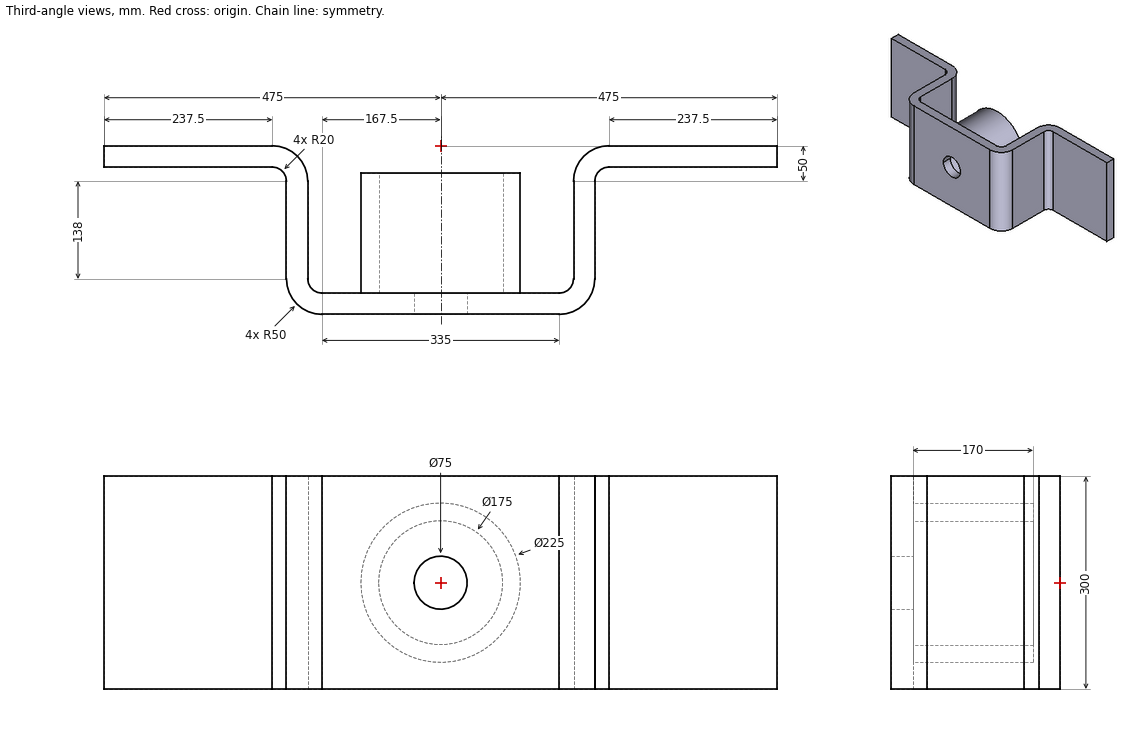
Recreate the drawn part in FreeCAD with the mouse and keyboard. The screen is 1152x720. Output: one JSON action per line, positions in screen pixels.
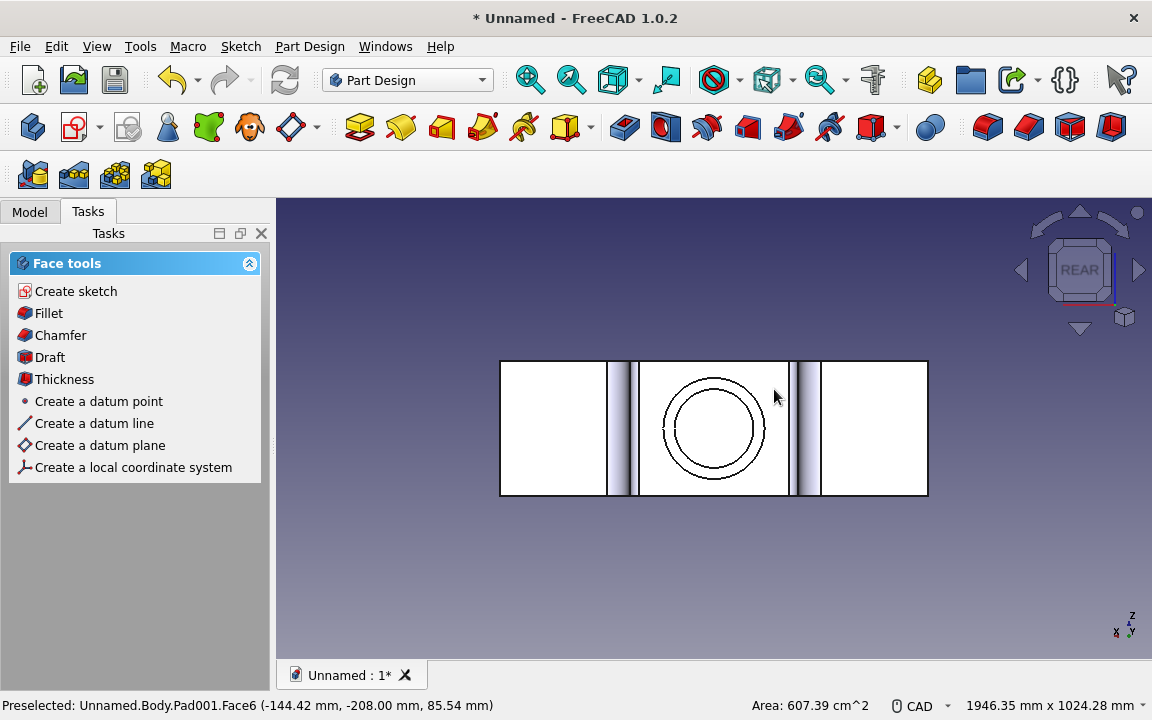
{"action": "left_click", "coordinate": [74, 128]}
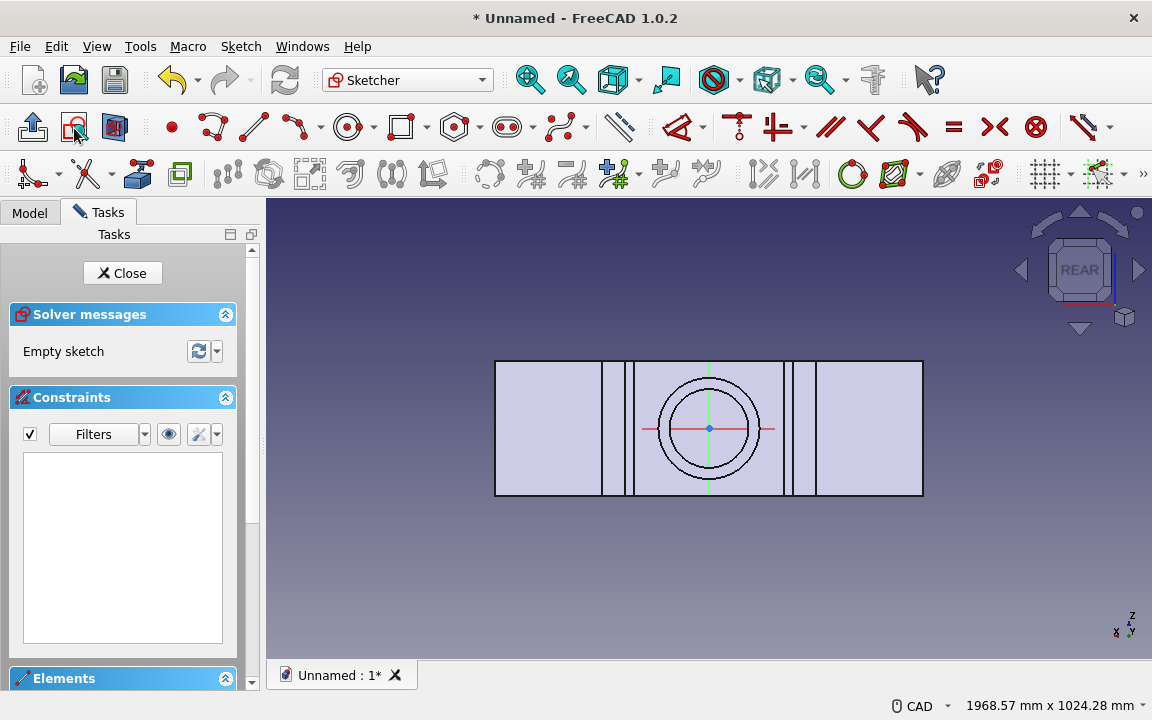
{"action": "scroll", "coordinate": [718, 429], "scroll_direction": "up", "scroll_amount": 11}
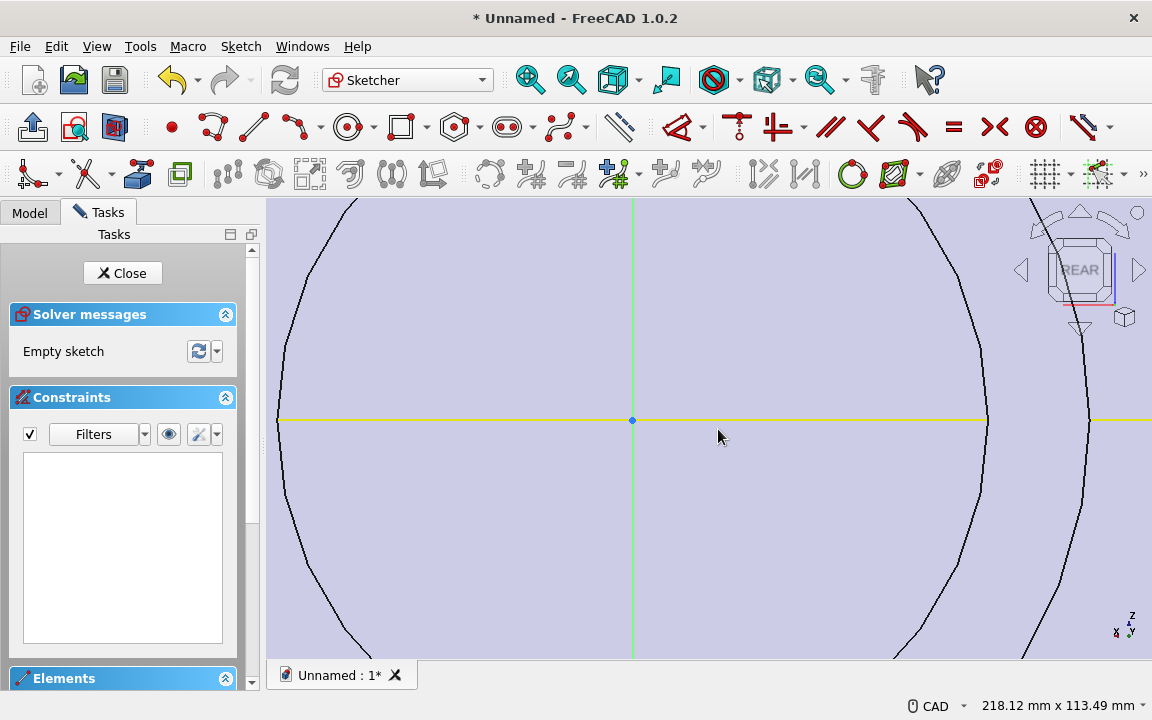
{"action": "key", "text": "g c"}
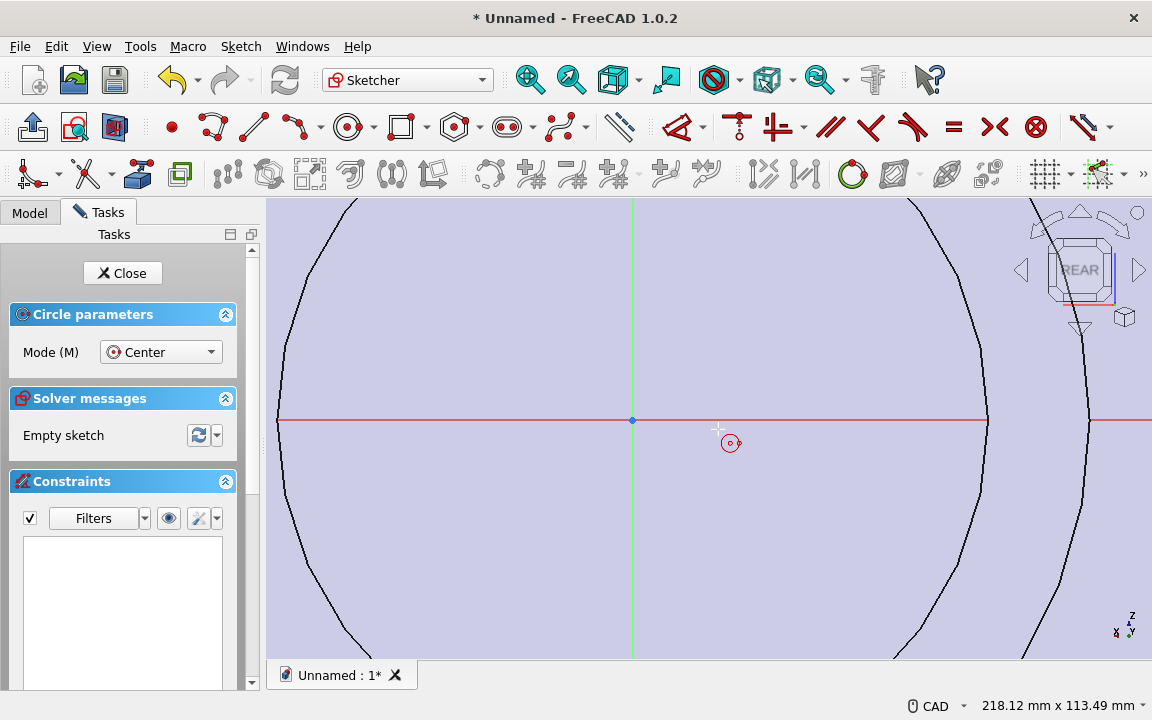
{"action": "left_click", "coordinate": [633, 420]}
{"action": "left_click", "coordinate": [740, 313]}
{"action": "key", "text": "Escape"}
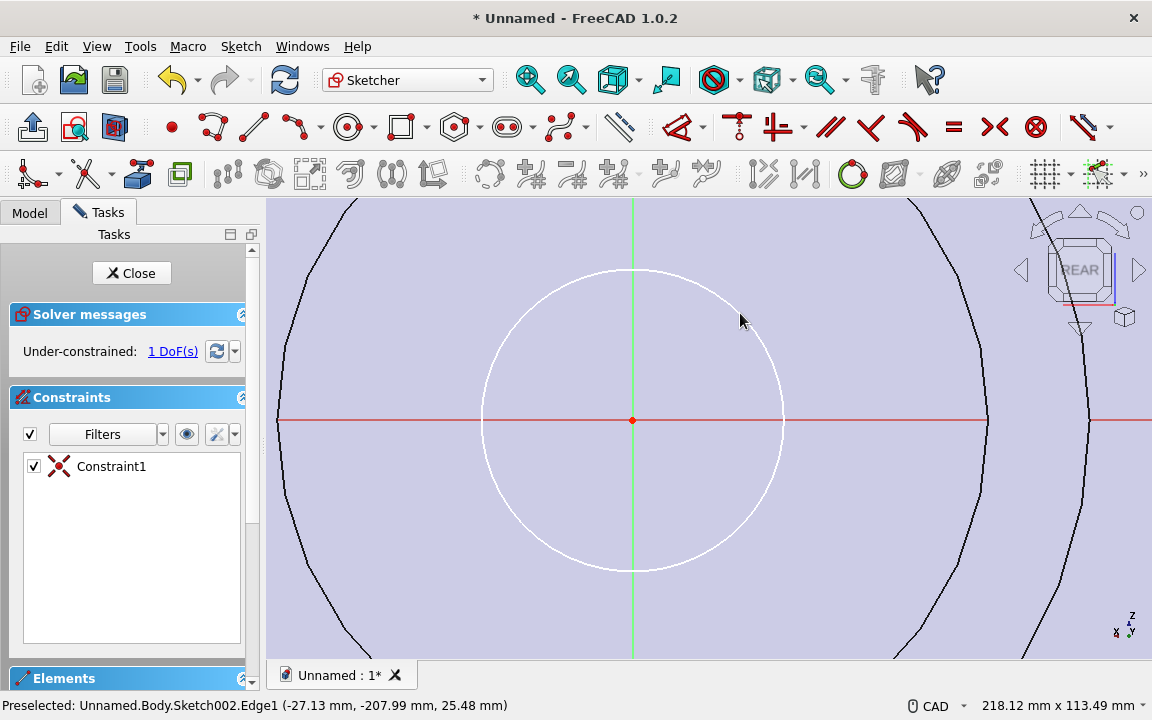
{"action": "key", "text": "d"}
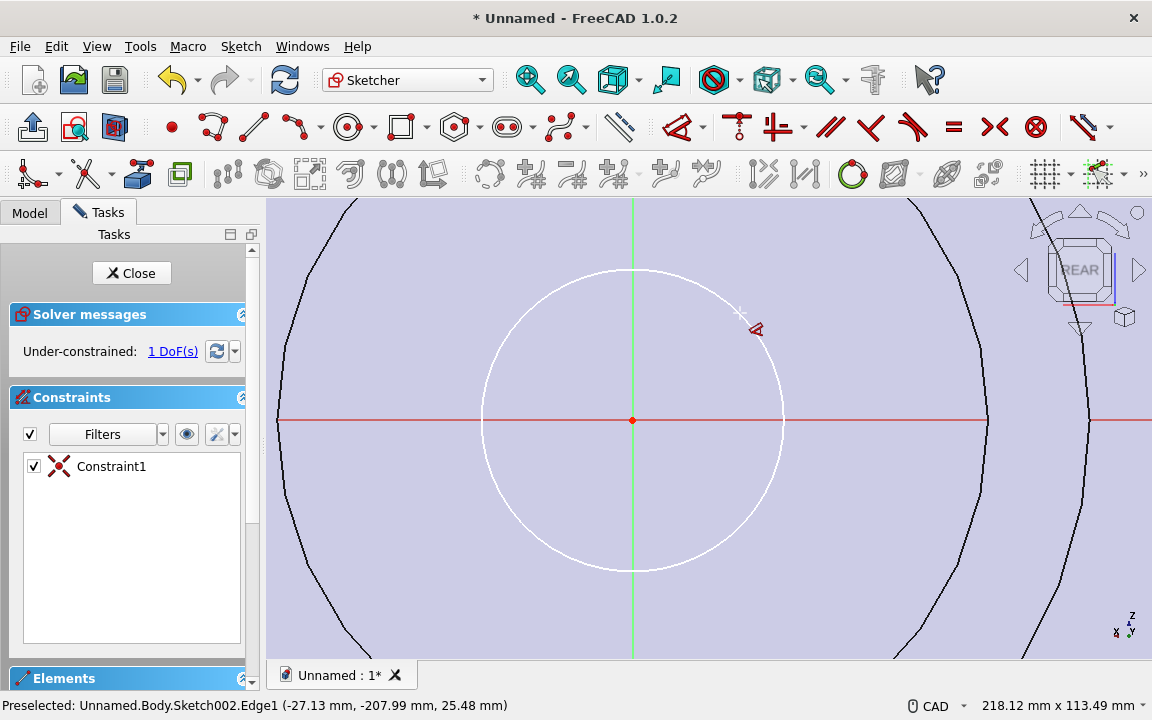
{"action": "left_click", "coordinate": [739, 313]}
{"action": "left_click", "coordinate": [762, 290]}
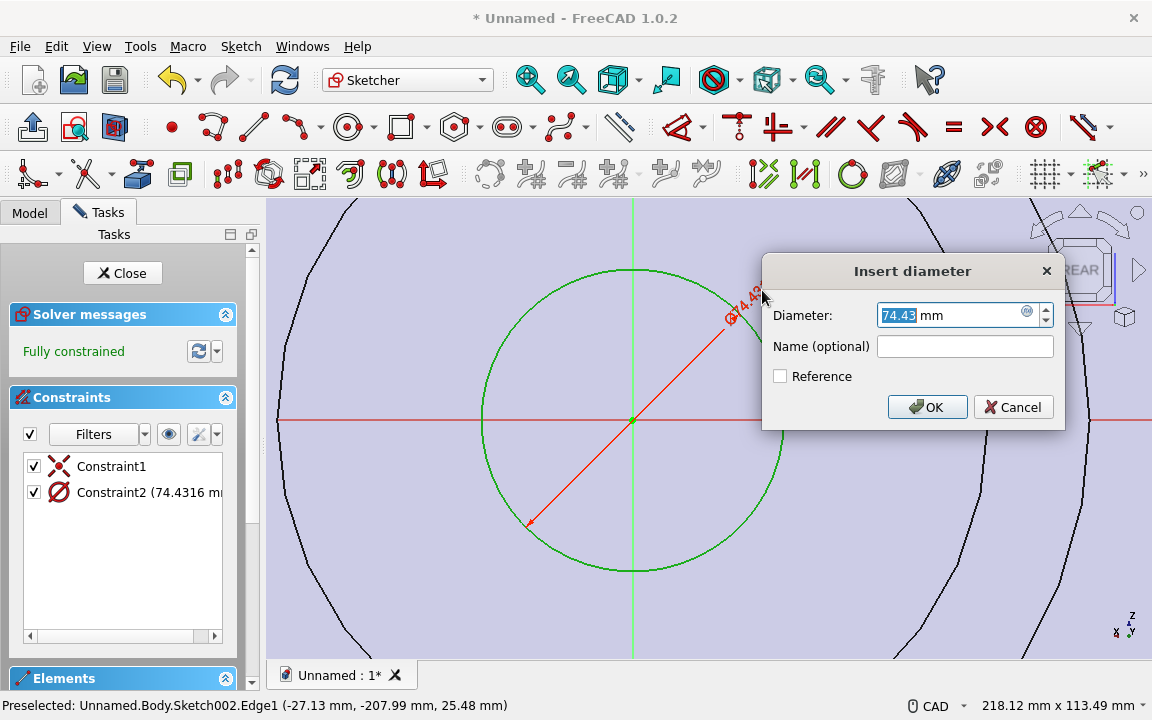
{"action": "type", "text": "75"}
{"action": "key", "text": "Return"}
{"action": "key", "text": "Escape"}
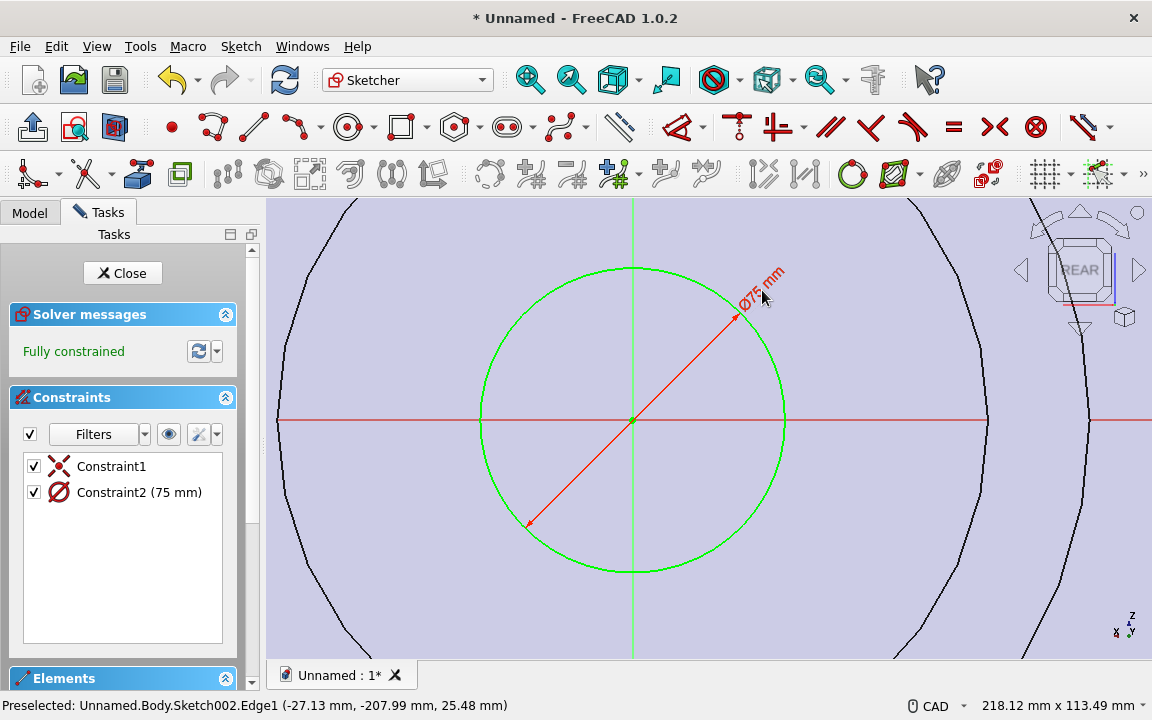
{"action": "left_click", "coordinate": [123, 273]}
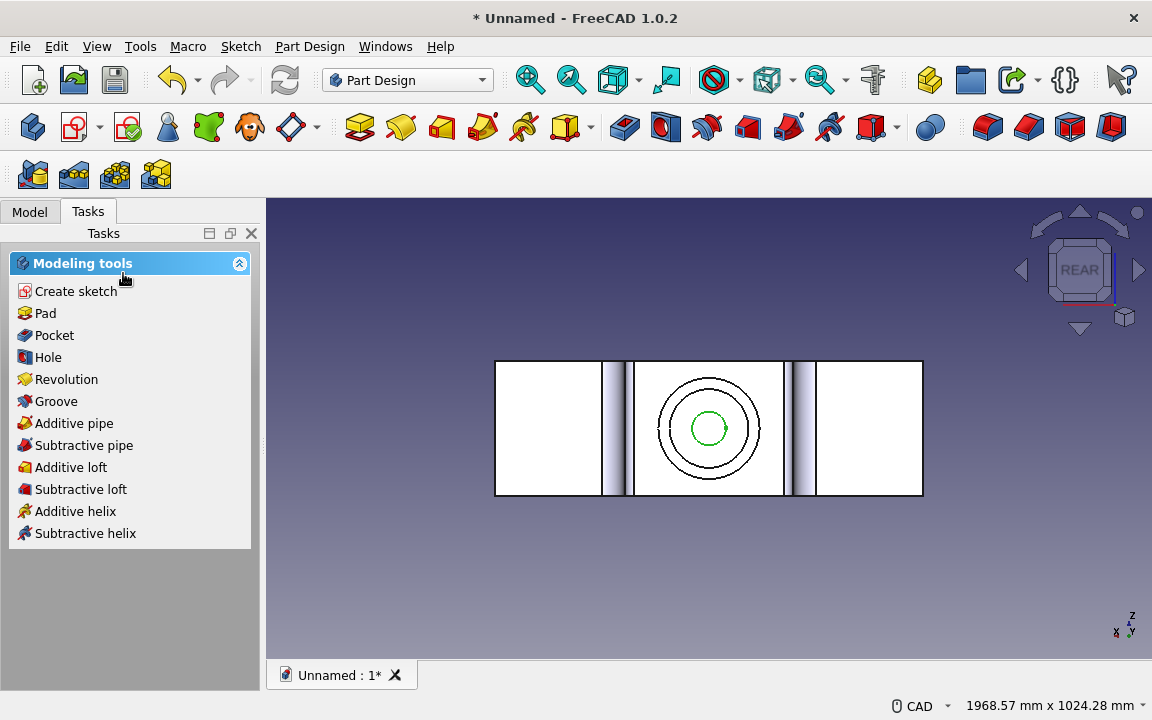
{"action": "left_click", "coordinate": [625, 128]}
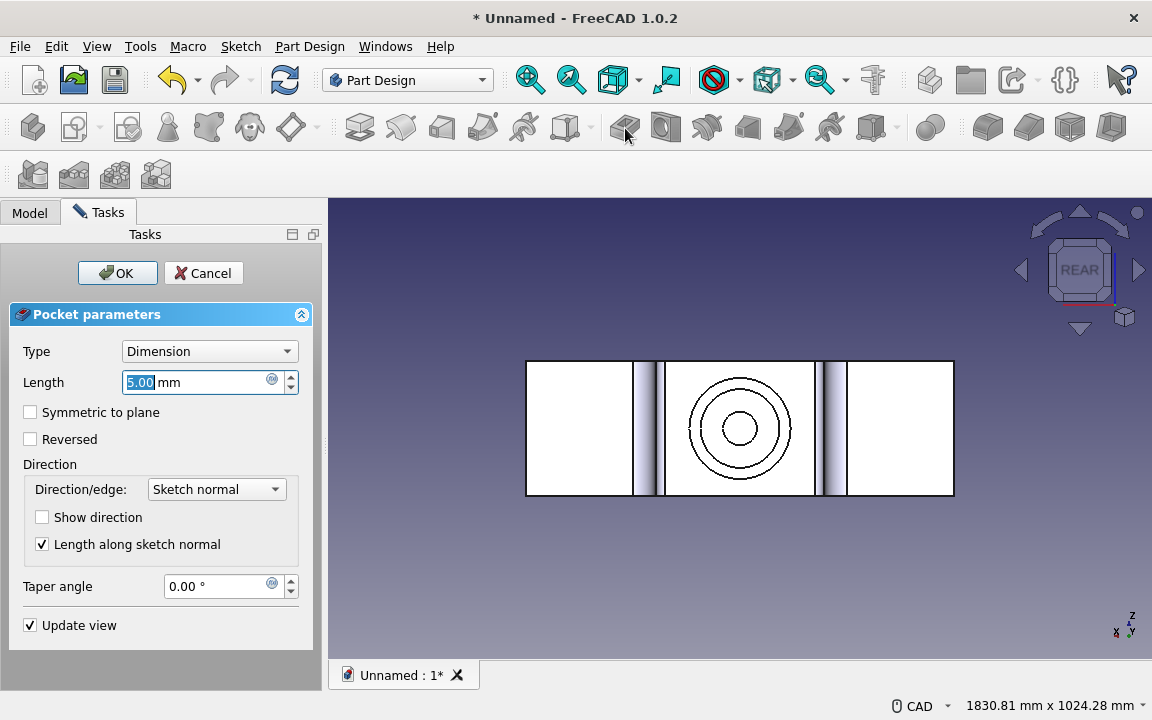
{"action": "left_click", "coordinate": [210, 352]}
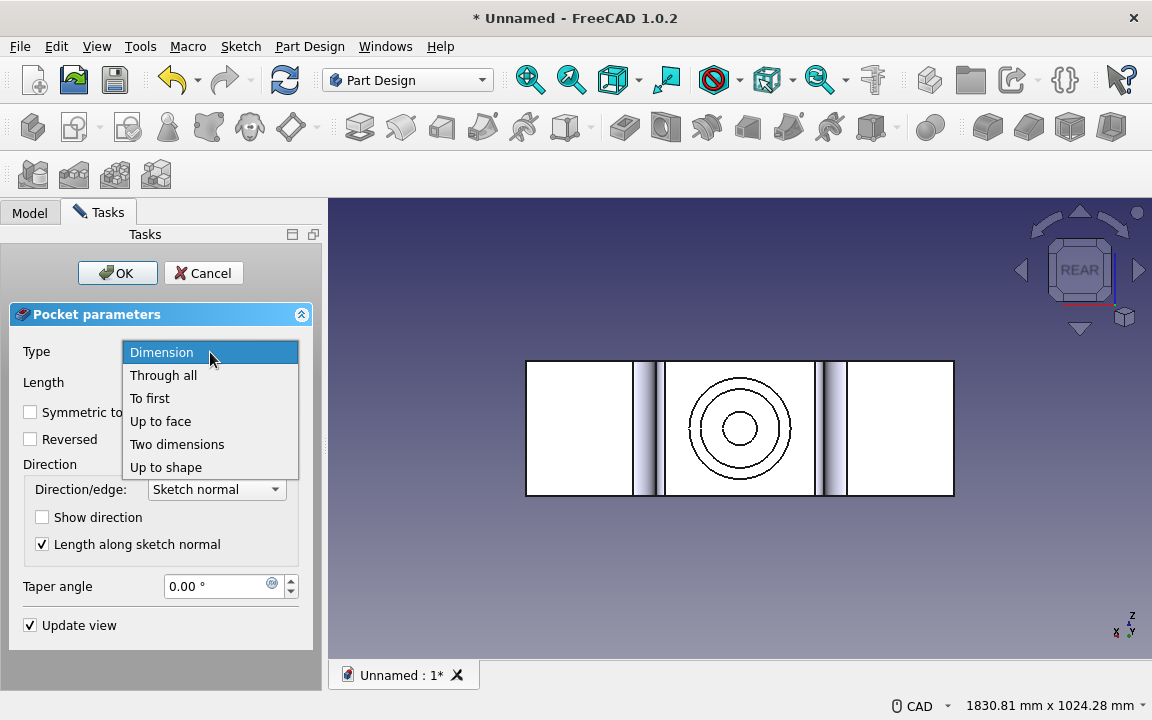
{"action": "left_click", "coordinate": [208, 398]}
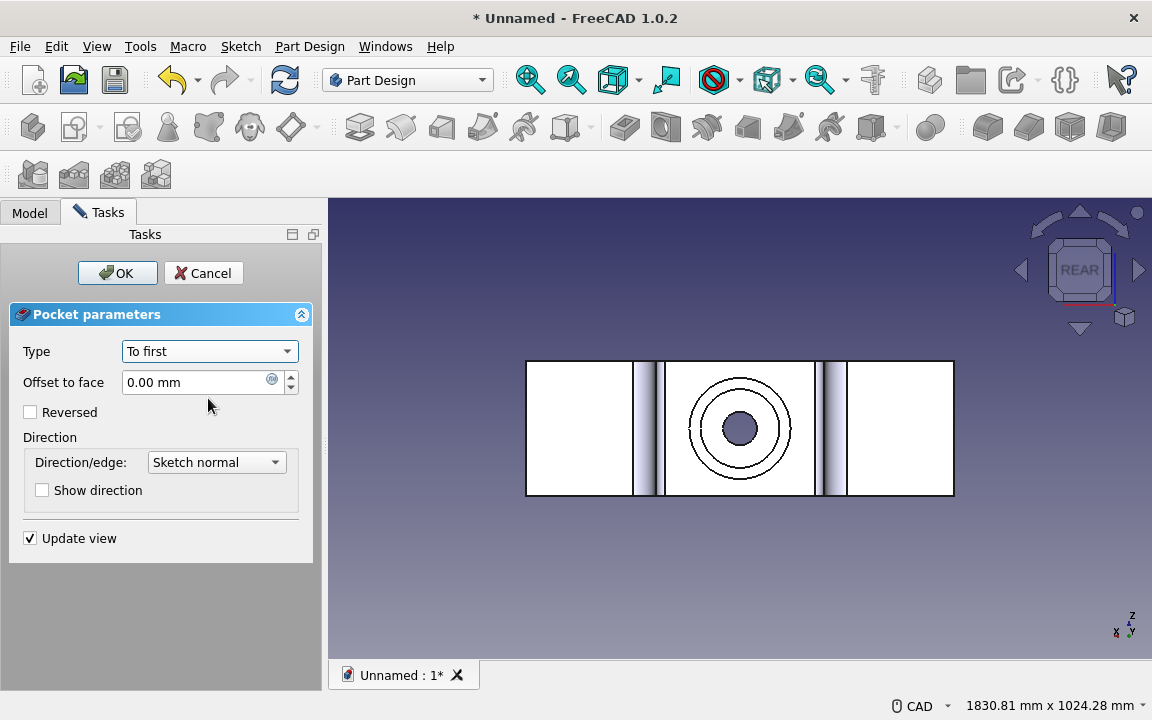
{"action": "left_click", "coordinate": [118, 273]}